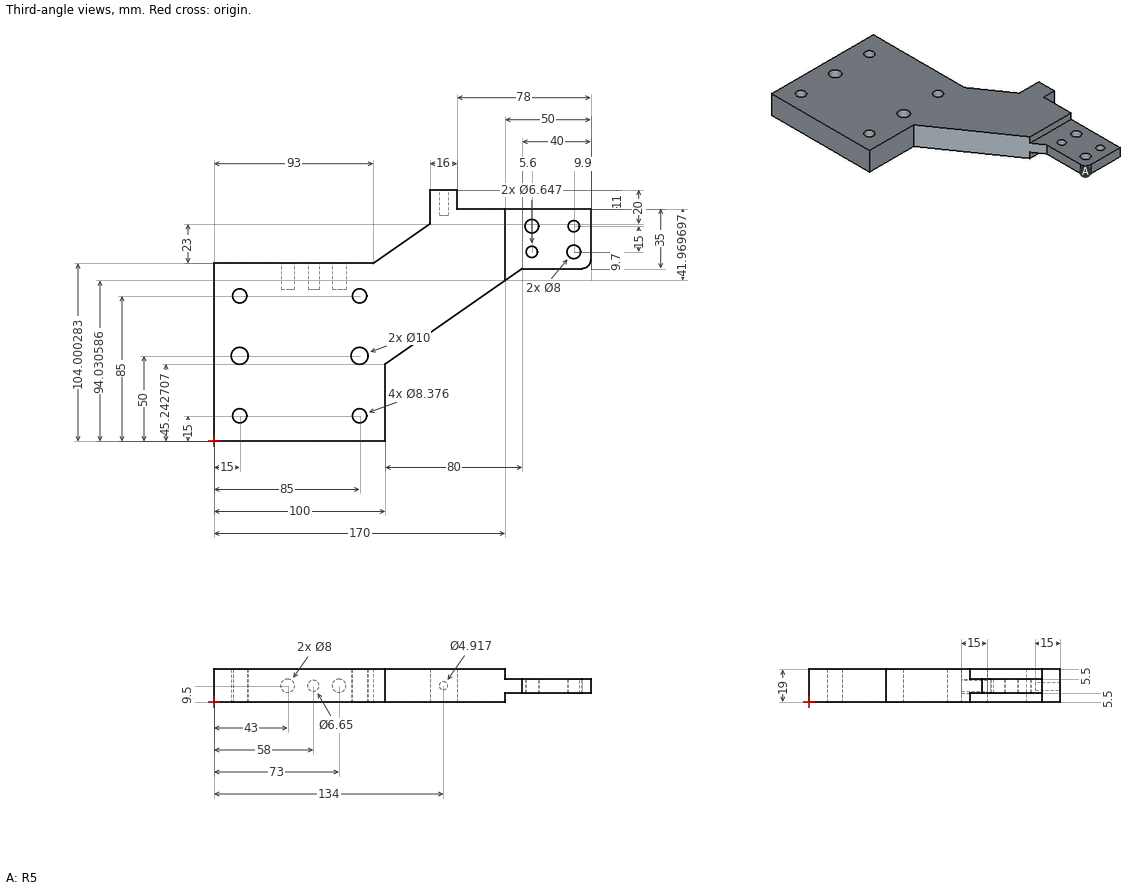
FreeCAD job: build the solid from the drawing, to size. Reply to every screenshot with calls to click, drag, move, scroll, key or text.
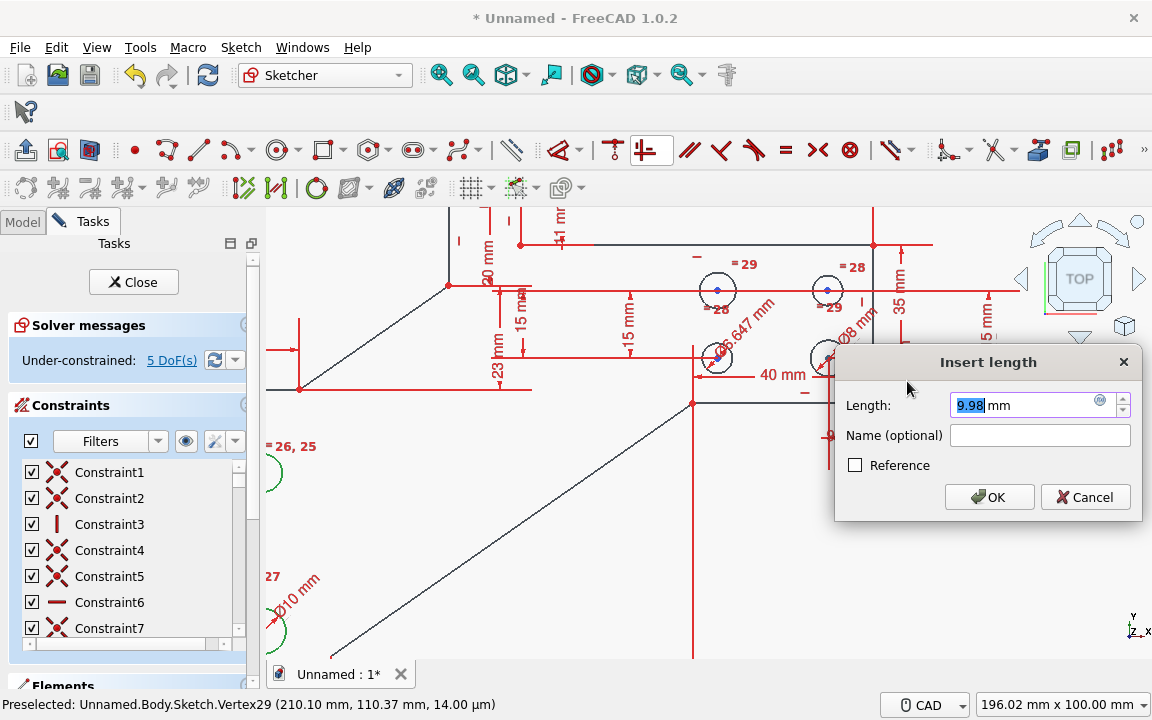
text(9.7)
key(Return)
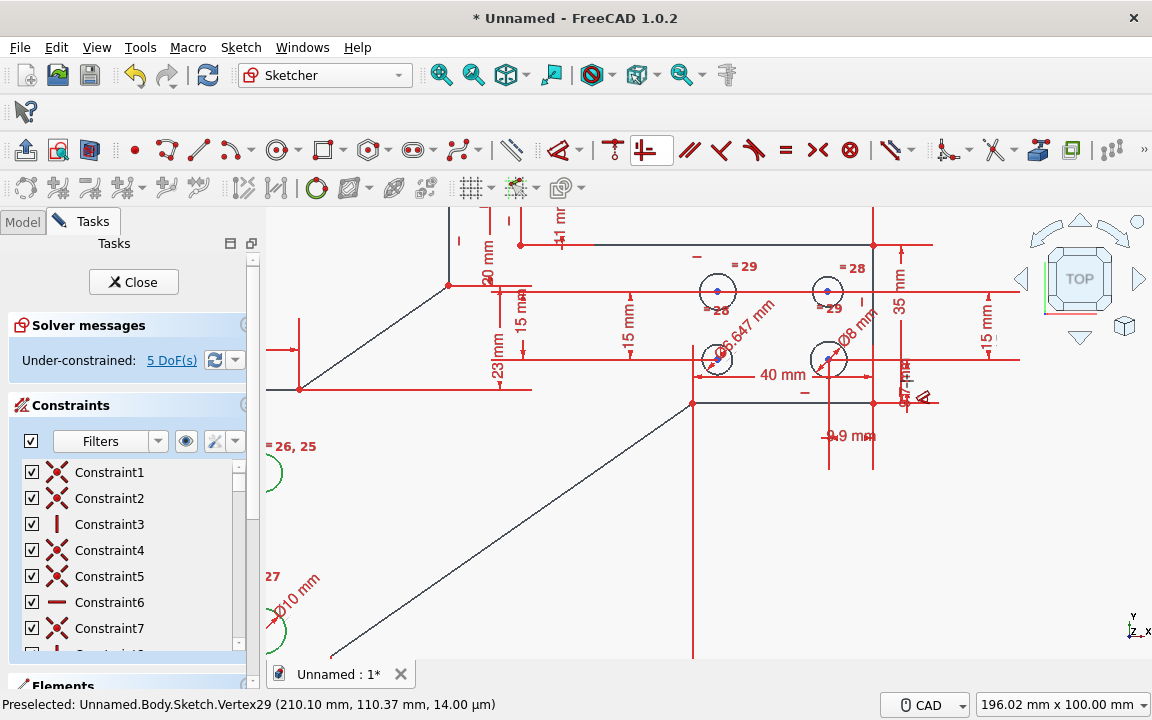
scroll(693, 403, up, 3)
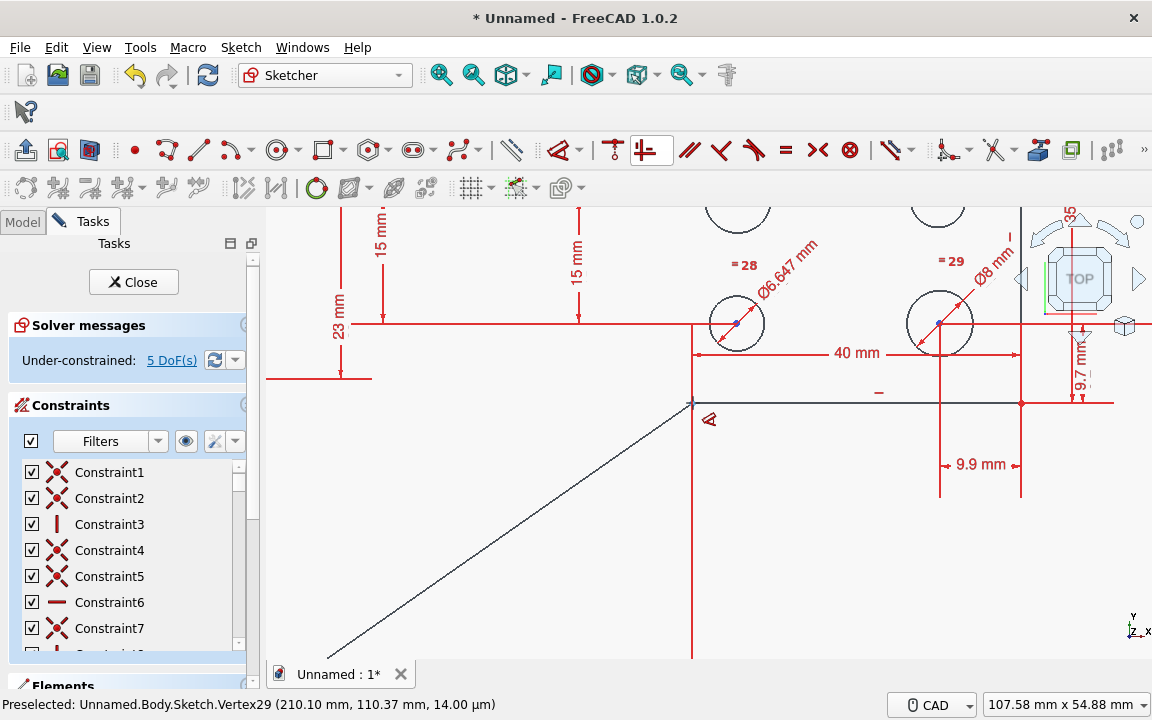
click(692, 403)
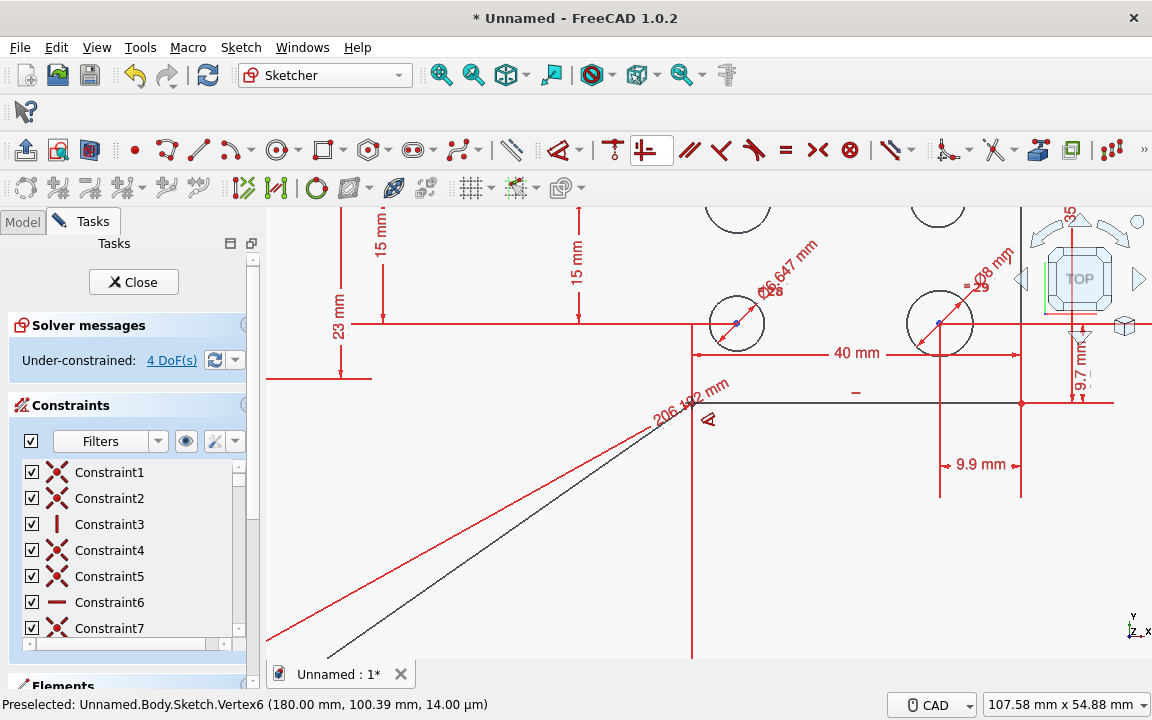
click(737, 324)
click(714, 290)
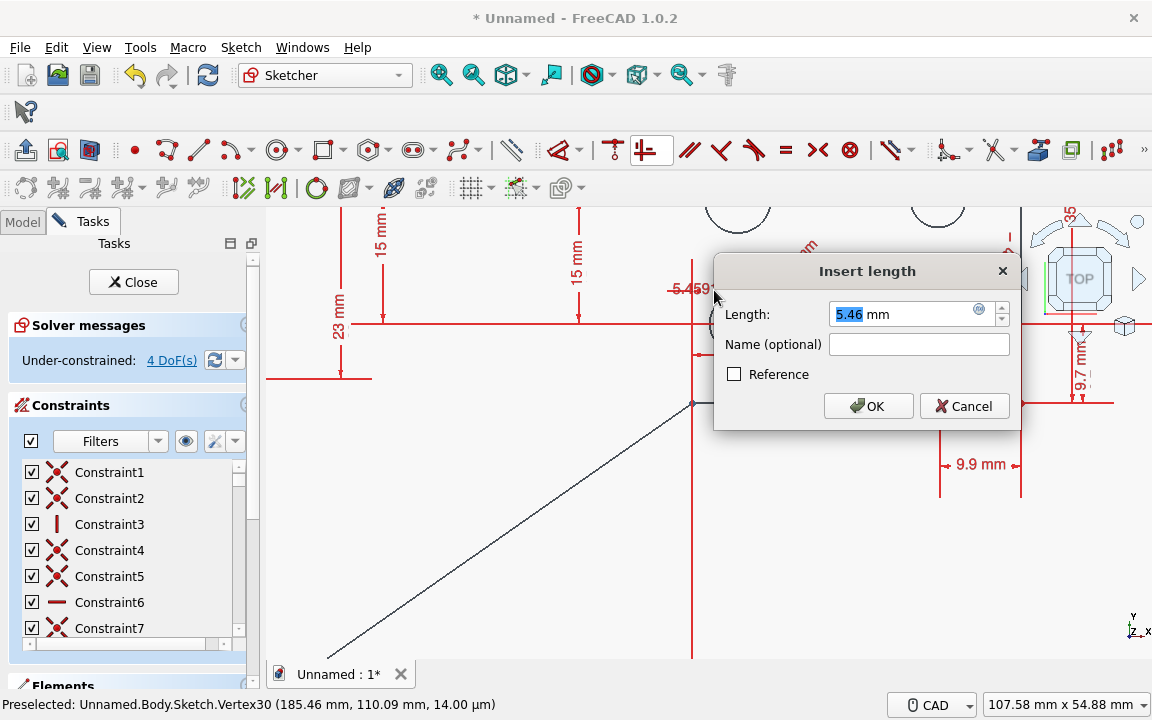
text(5.6)
key(Return)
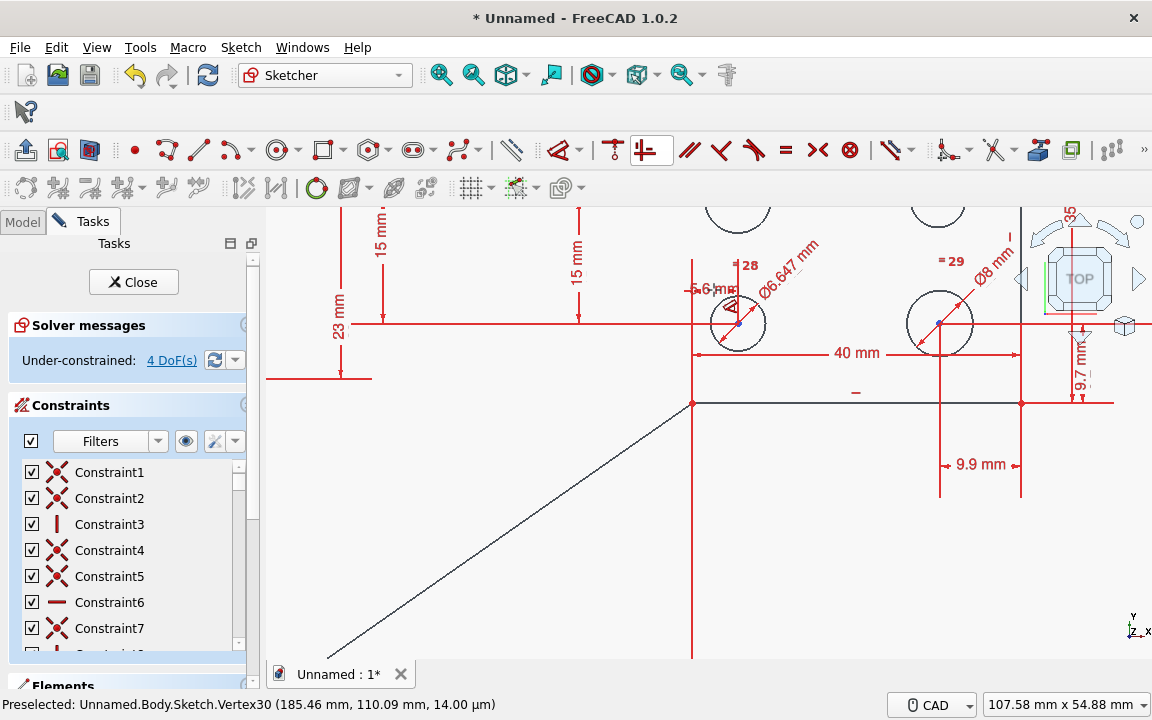
scroll(812, 370, down, 7)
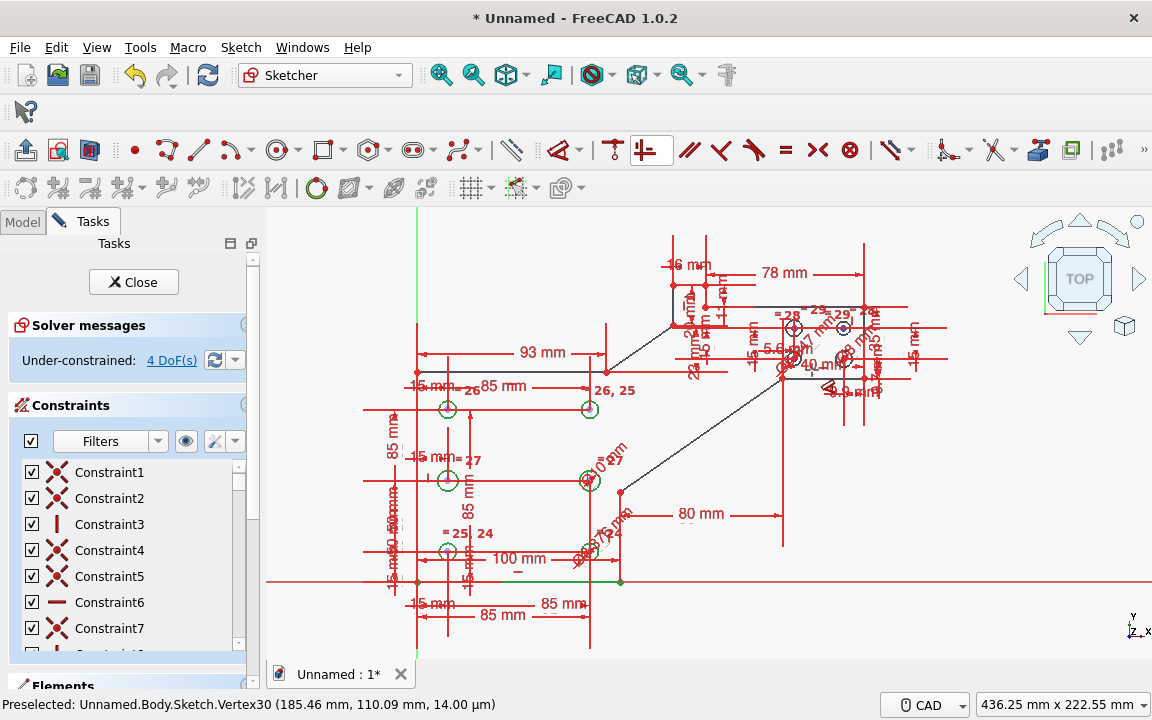
scroll(864, 307, up, 4)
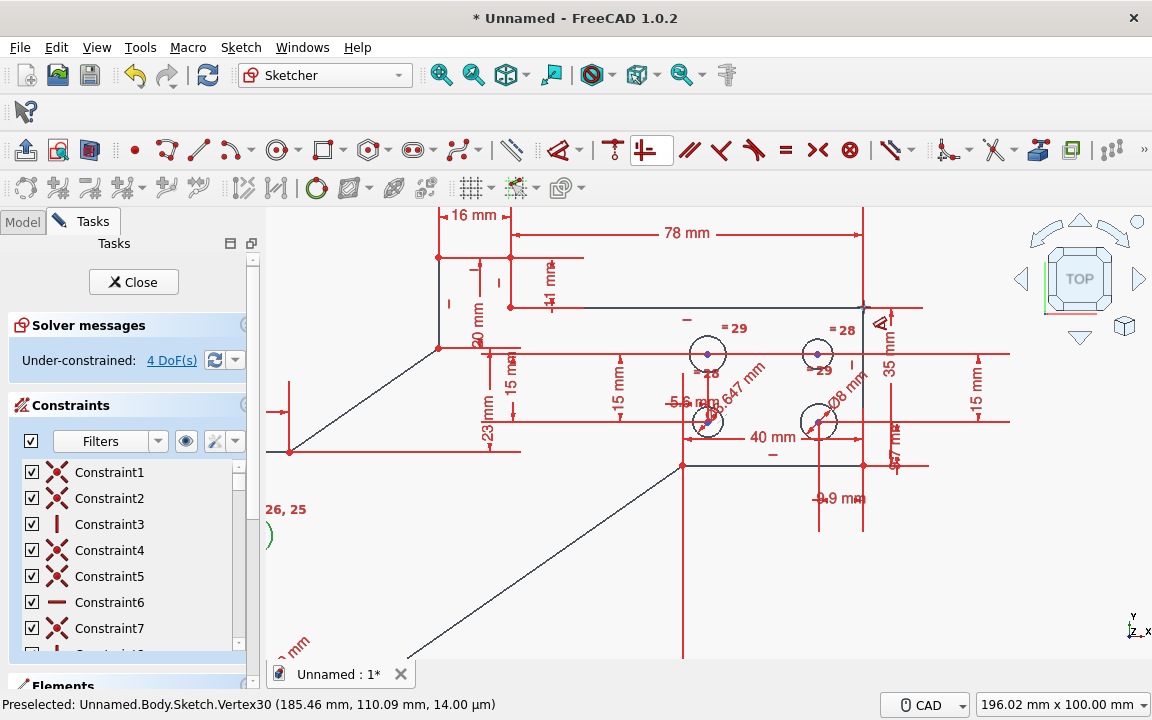
click(863, 308)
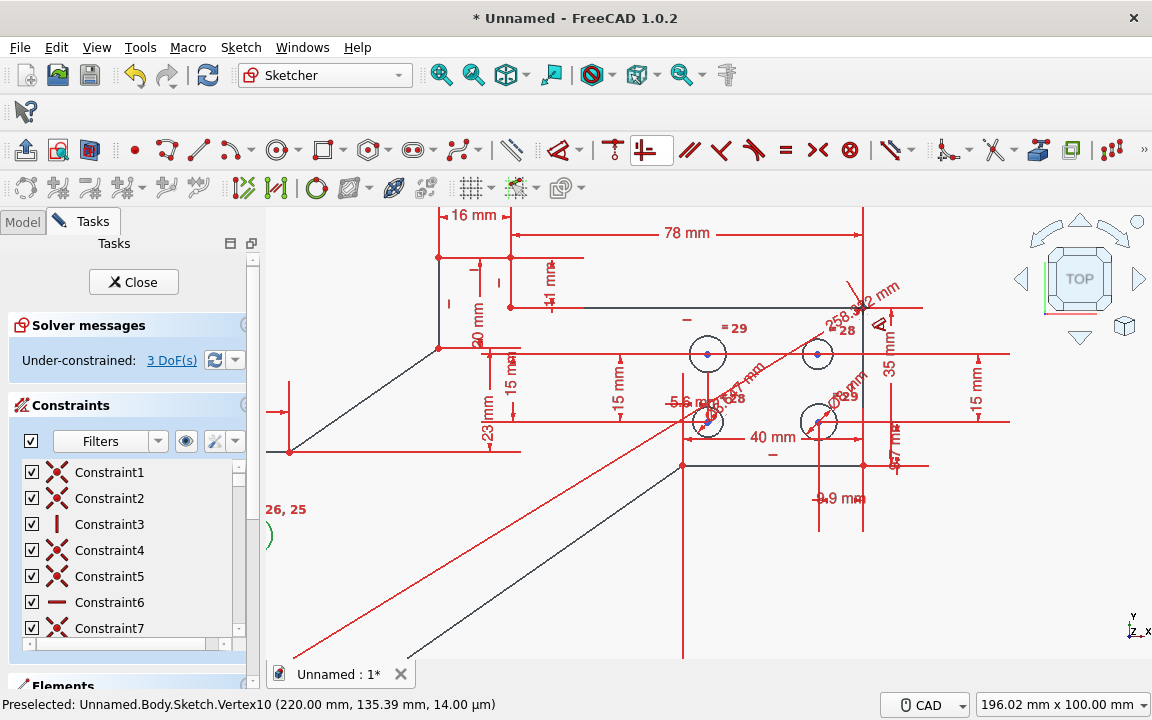
click(818, 354)
click(841, 274)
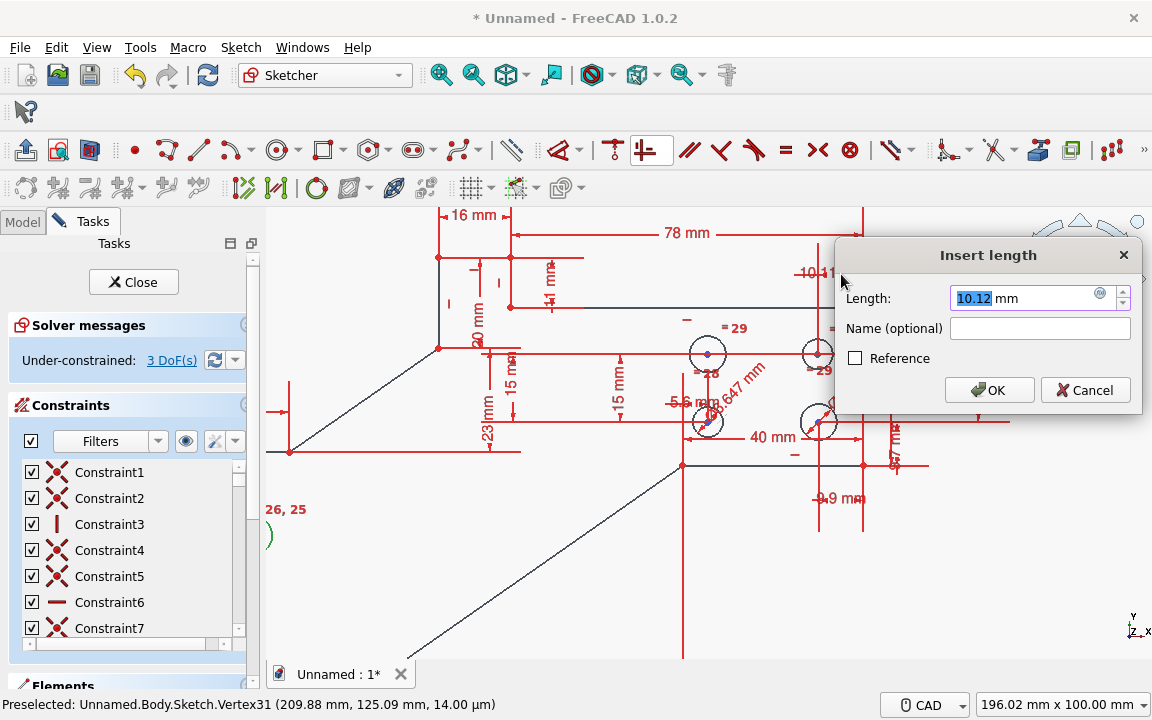
text(9.9)
key(Return)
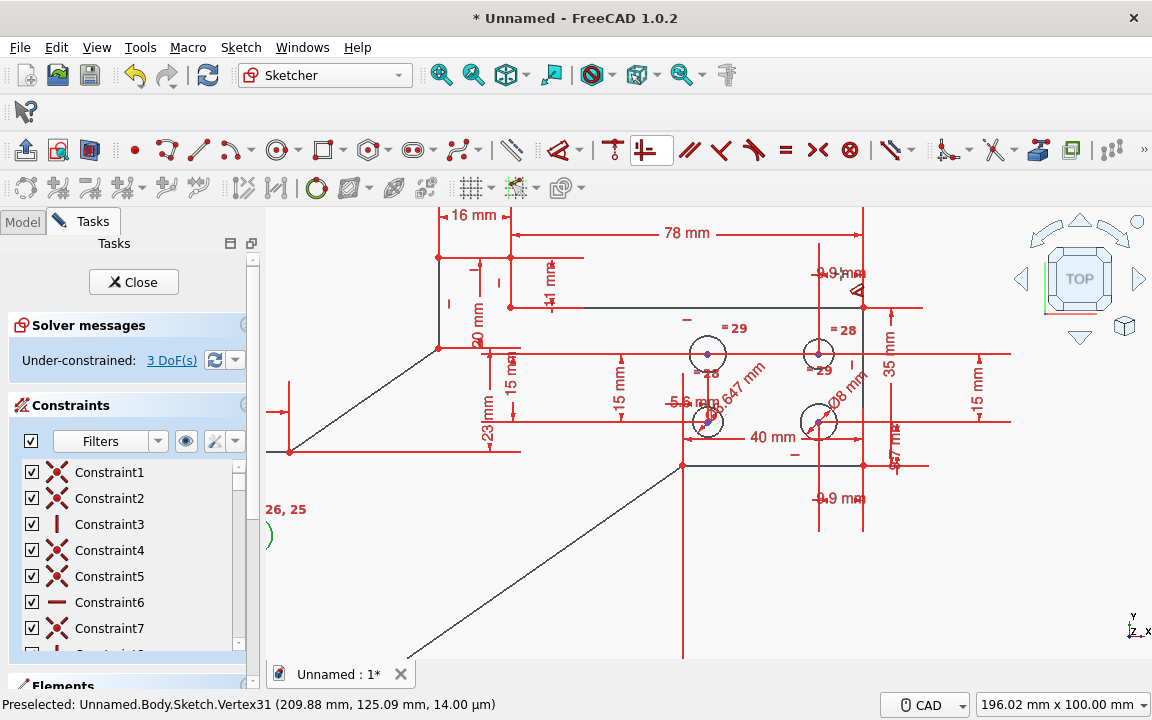
scroll(683, 466, up, 3)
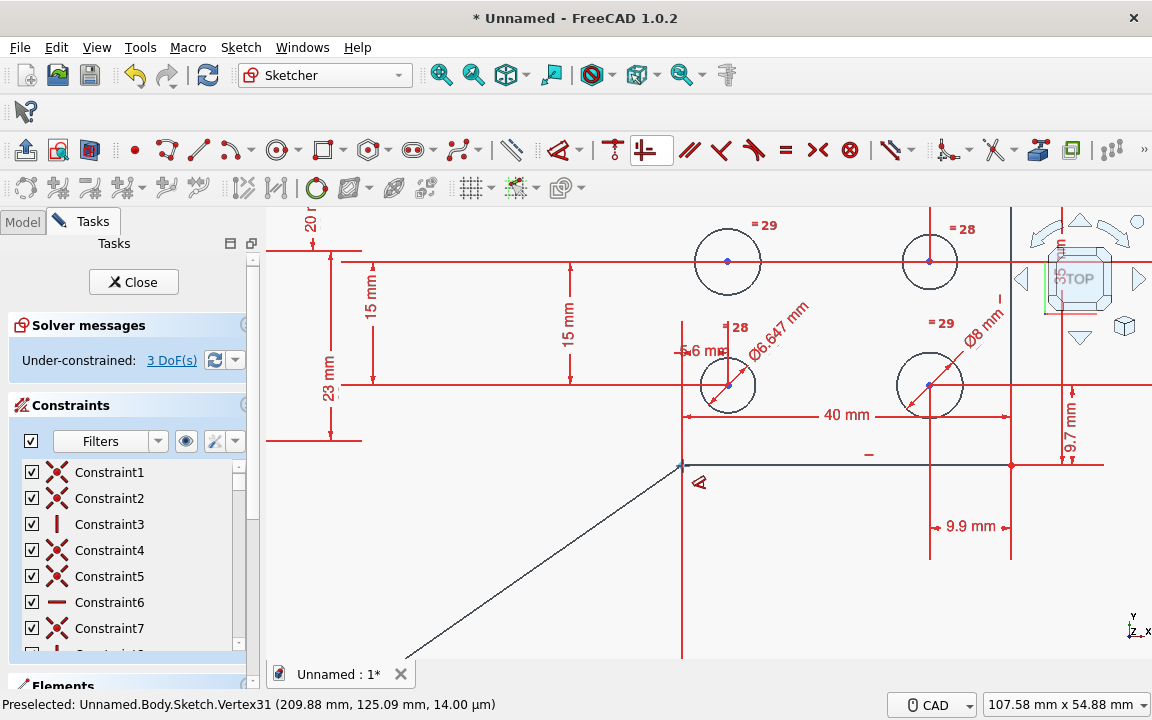
click(682, 465)